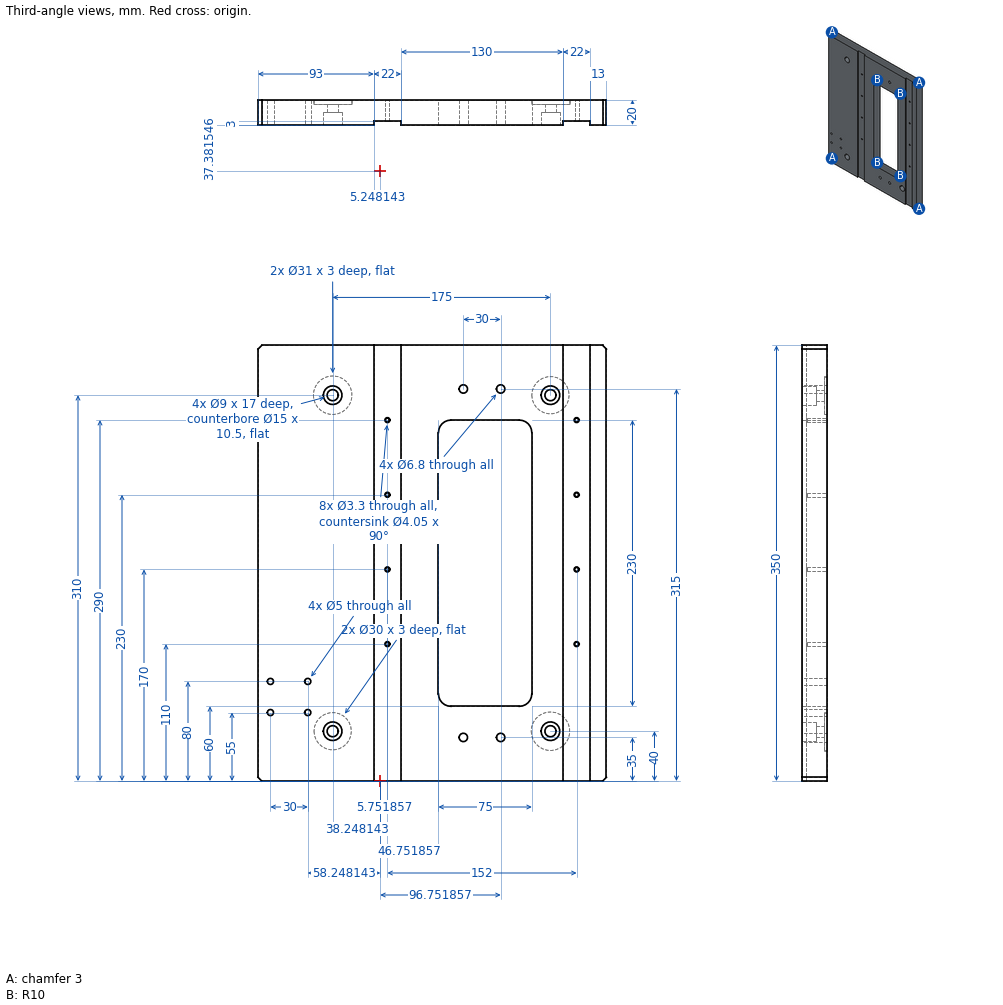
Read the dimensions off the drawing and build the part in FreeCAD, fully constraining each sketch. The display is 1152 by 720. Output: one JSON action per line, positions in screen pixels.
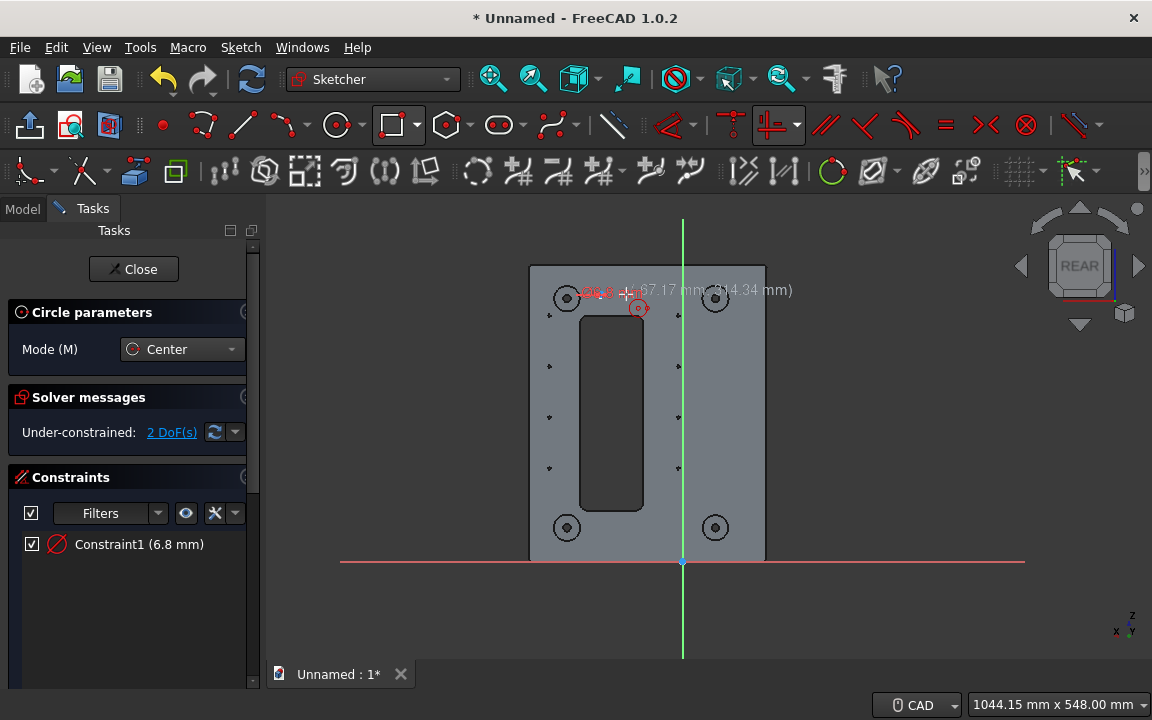
{"action": "left_click", "coordinate": [626, 294]}
{"action": "mouse_move", "coordinate": [628, 292]}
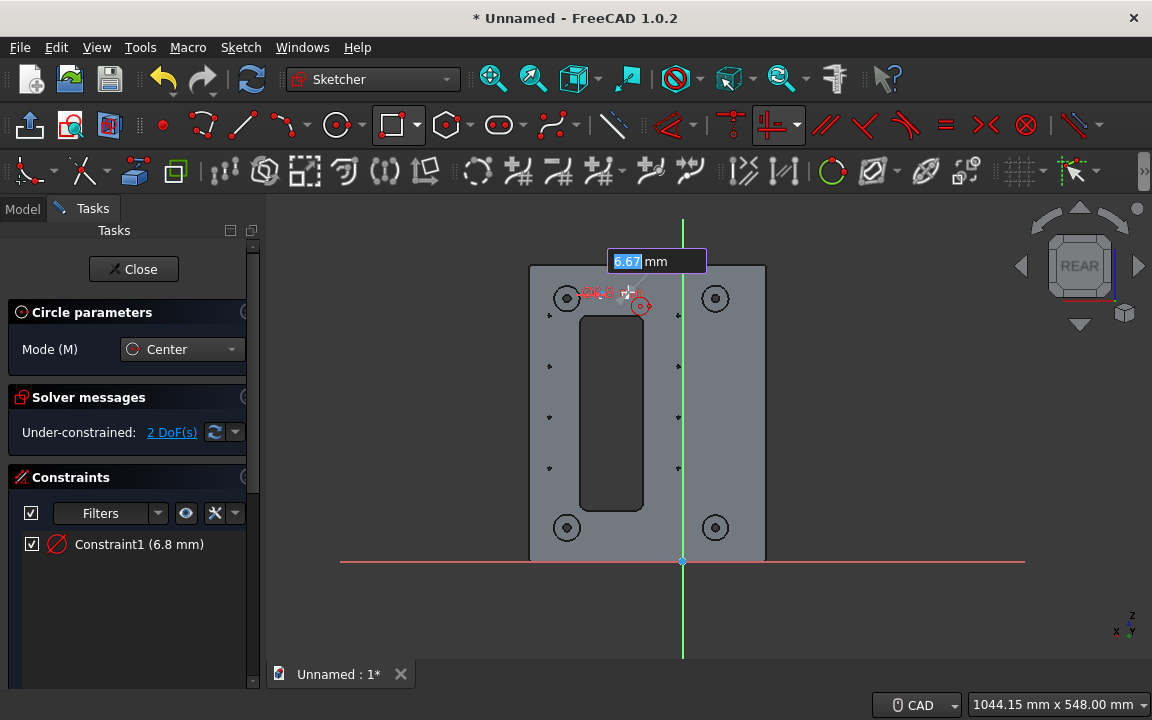
{"action": "type", "text": "6.8"}
{"action": "key", "text": "Return"}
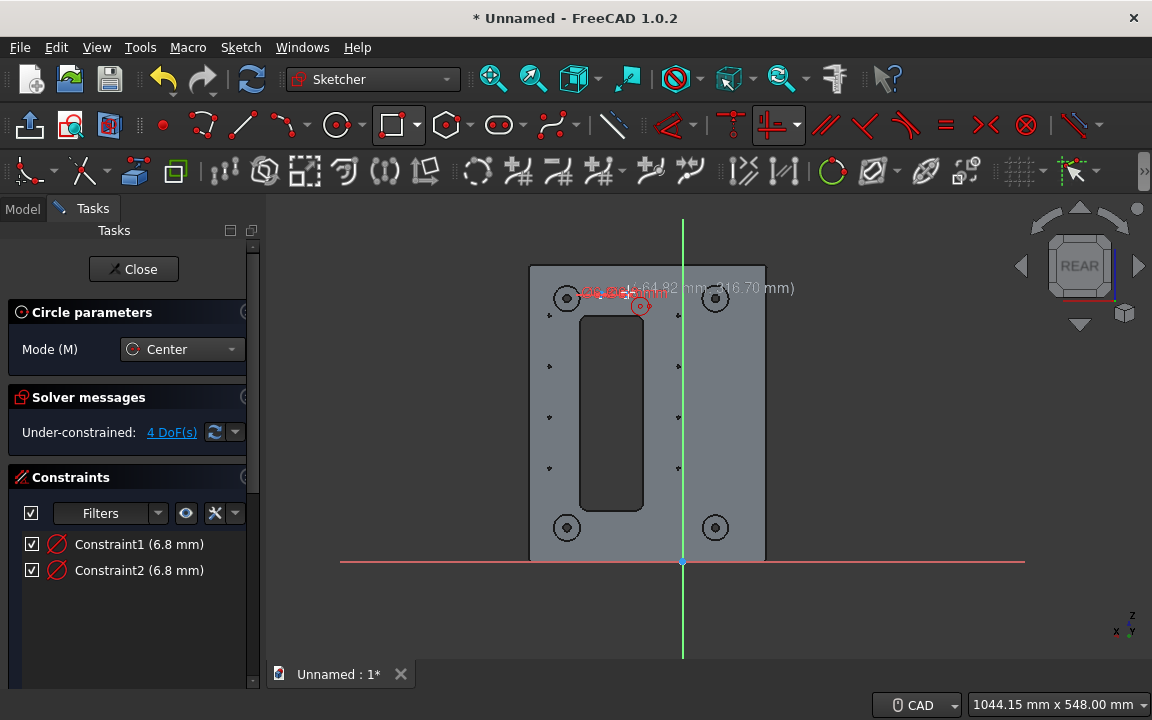
{"action": "scroll", "coordinate": [601, 532], "scroll_direction": "up", "scroll_amount": 11}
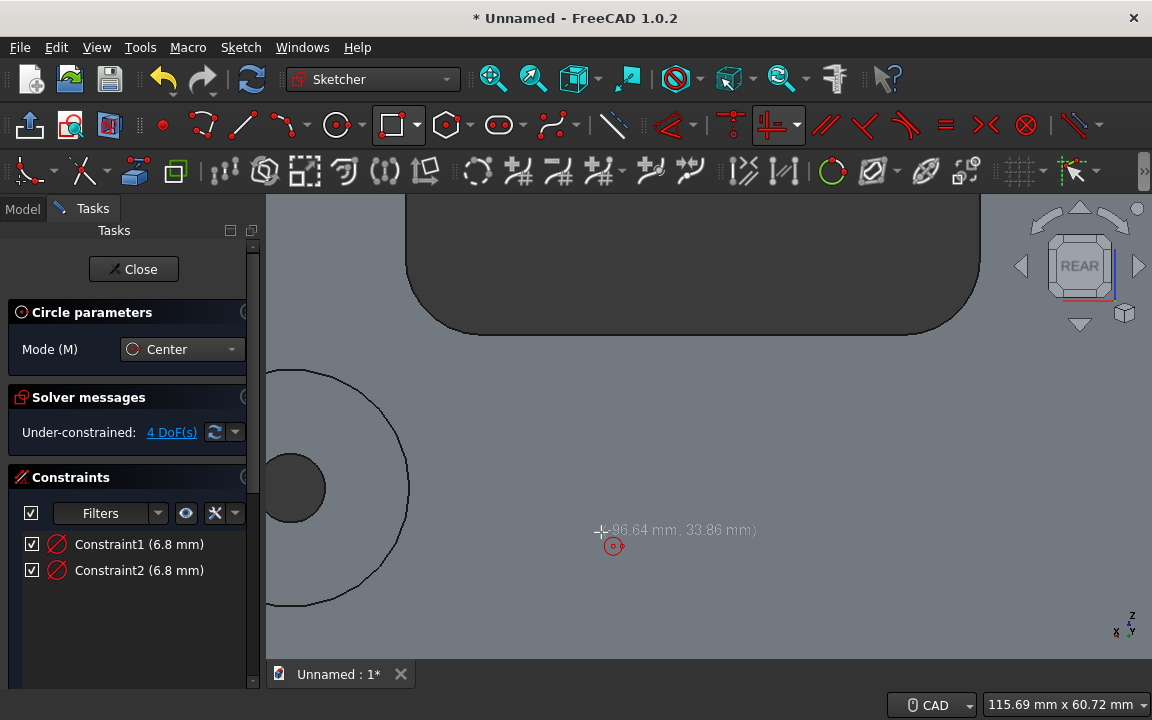
{"action": "scroll", "coordinate": [601, 533], "scroll_direction": "down", "scroll_amount": 11}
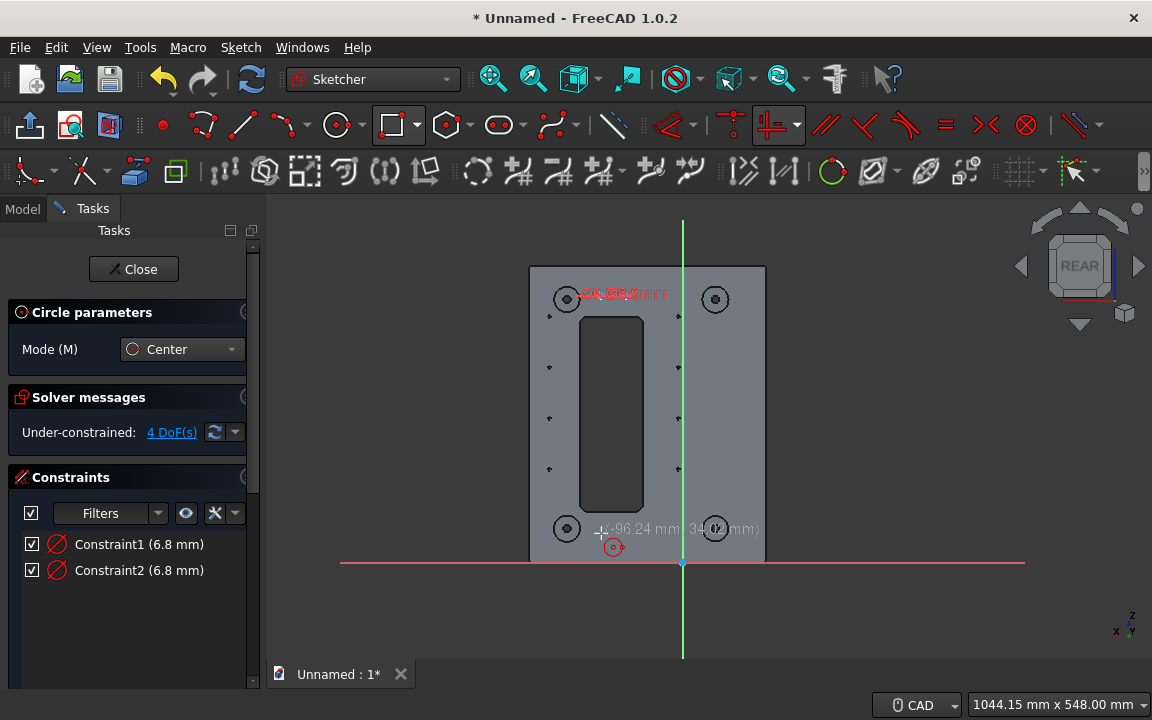
{"action": "left_click", "coordinate": [601, 533]}
{"action": "mouse_move", "coordinate": [603, 531]}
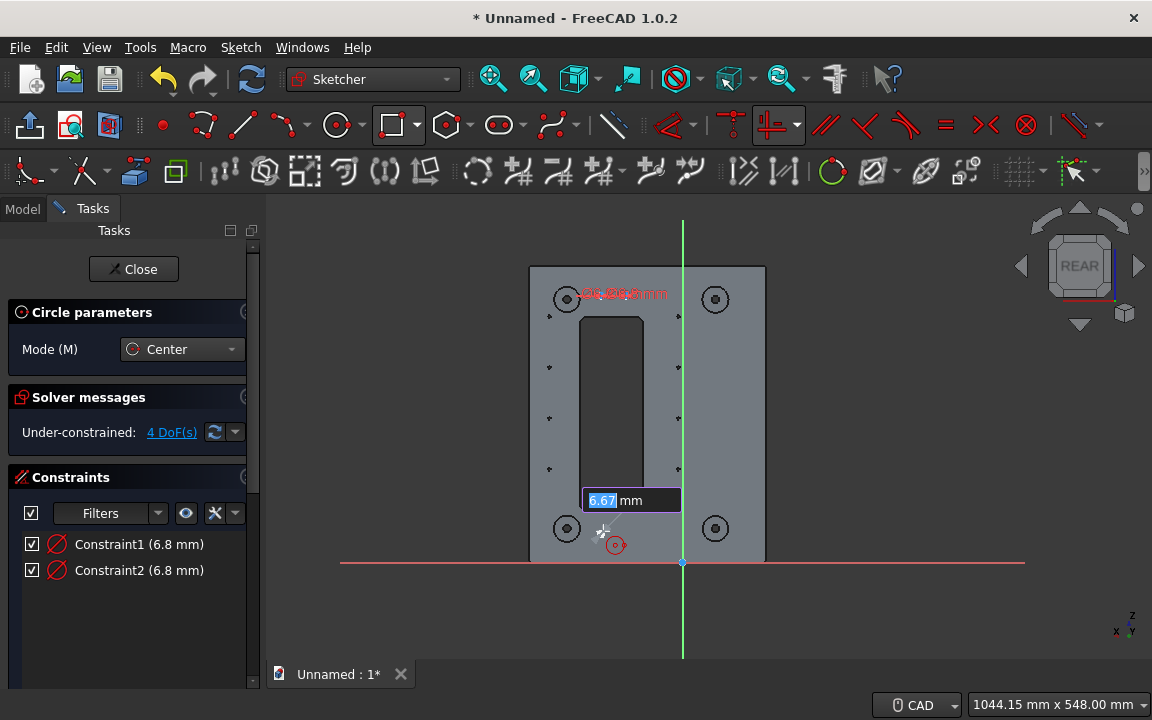
{"action": "type", "text": "6.8"}
{"action": "key", "text": "Return"}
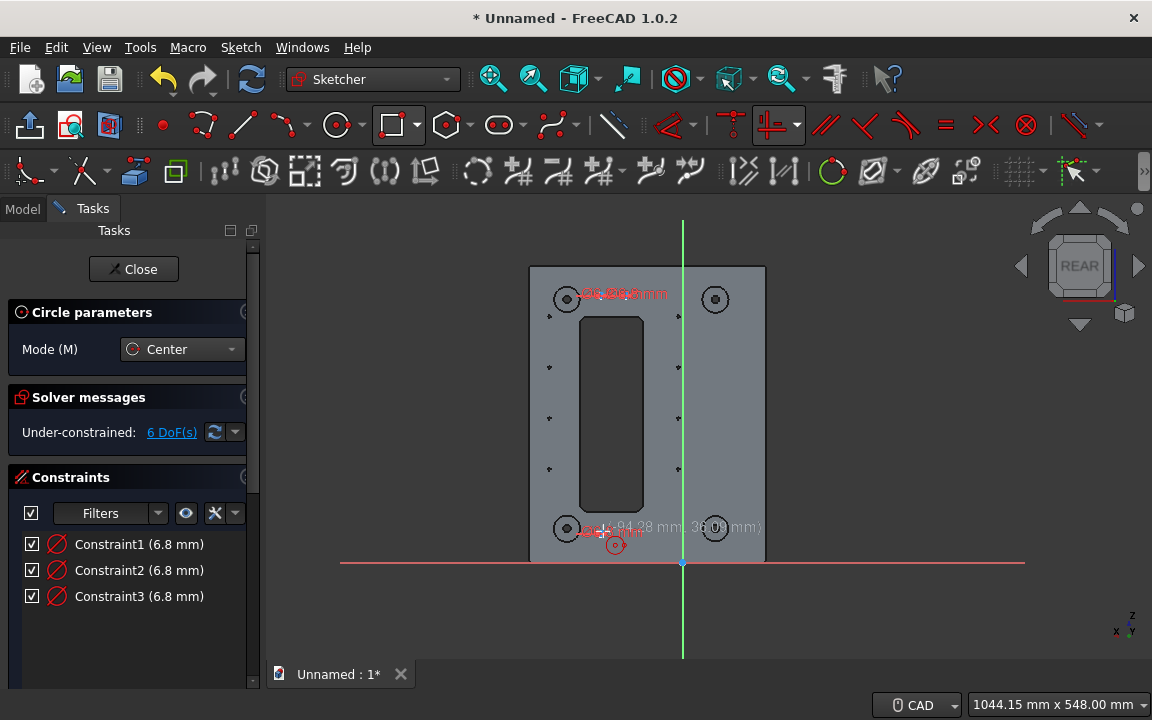
{"action": "scroll", "coordinate": [626, 533], "scroll_direction": "up", "scroll_amount": 11}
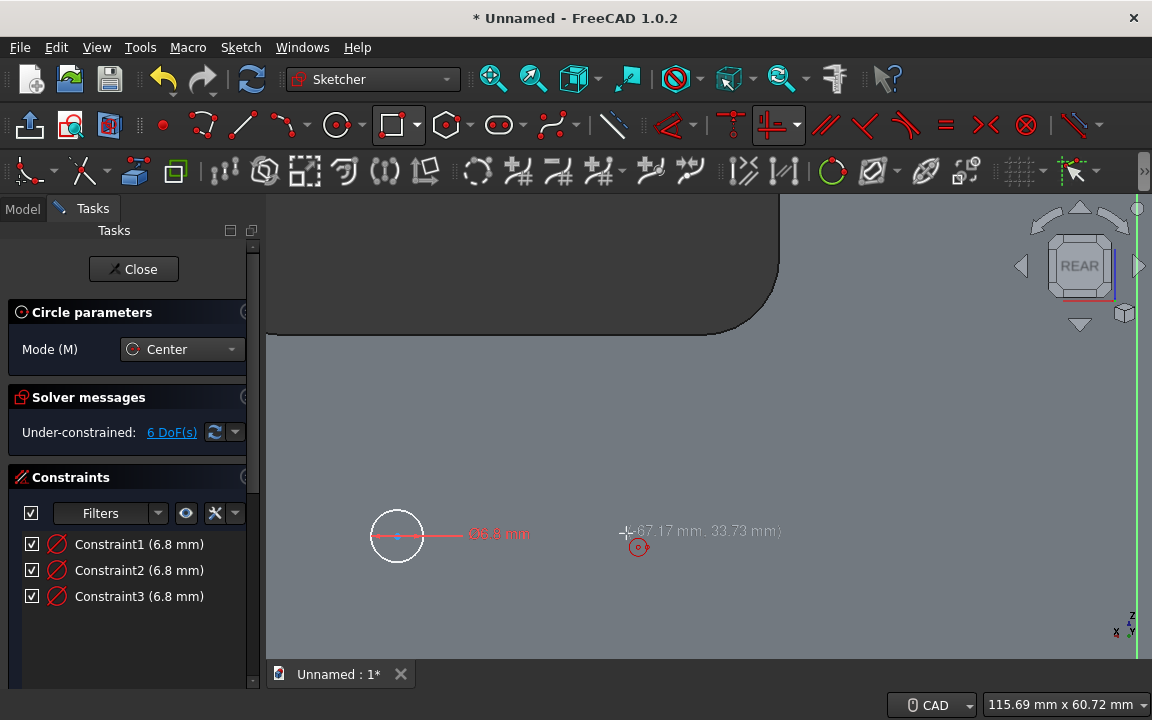
{"action": "scroll", "coordinate": [626, 533], "scroll_direction": "down", "scroll_amount": 11}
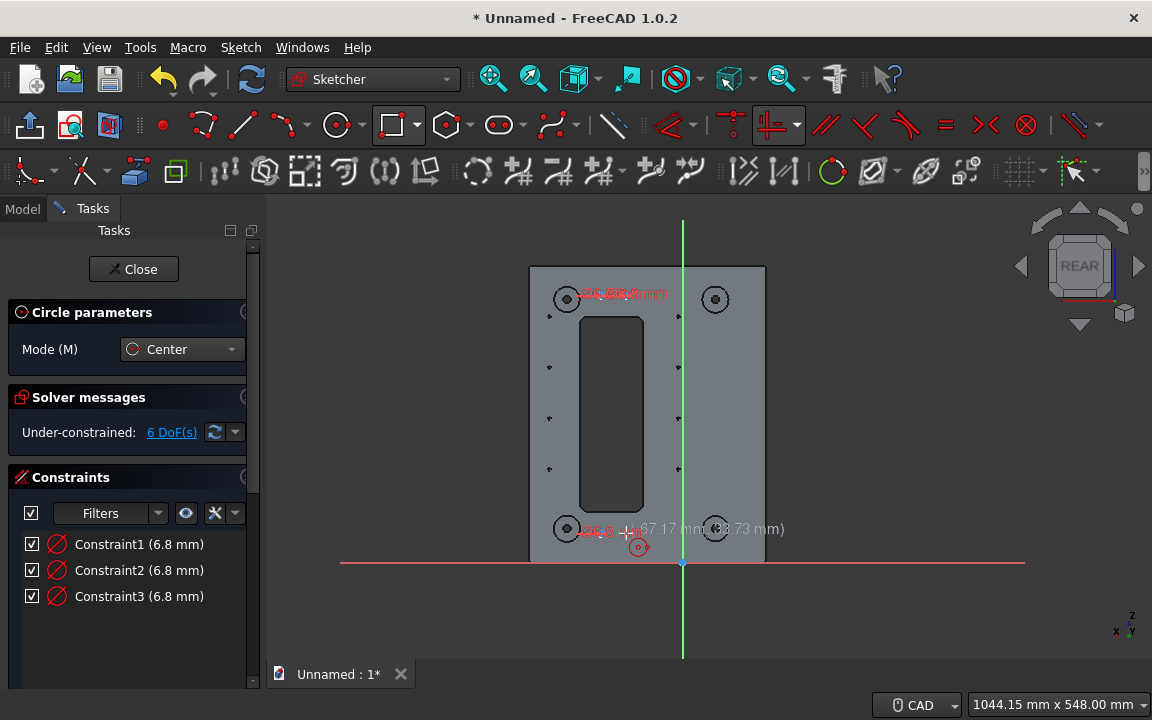
{"action": "left_click", "coordinate": [626, 533]}
{"action": "mouse_move", "coordinate": [628, 531]}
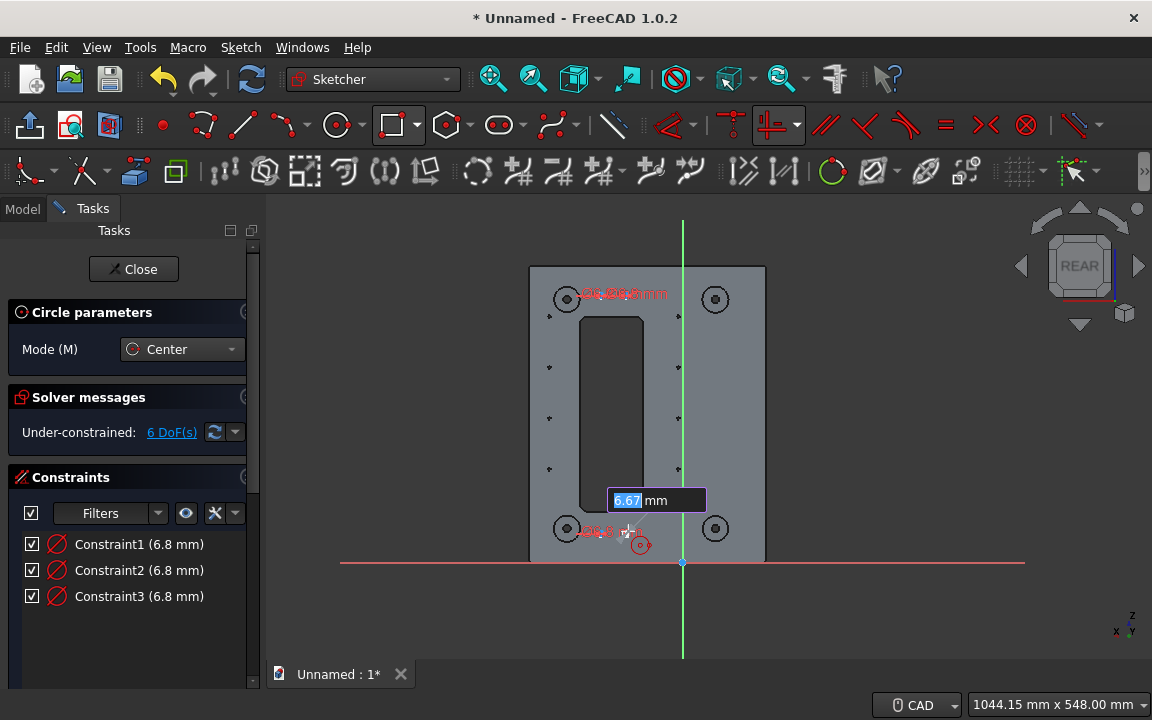
{"action": "type", "text": "6.8"}
{"action": "key", "text": "Return"}
{"action": "key", "text": "Escape"}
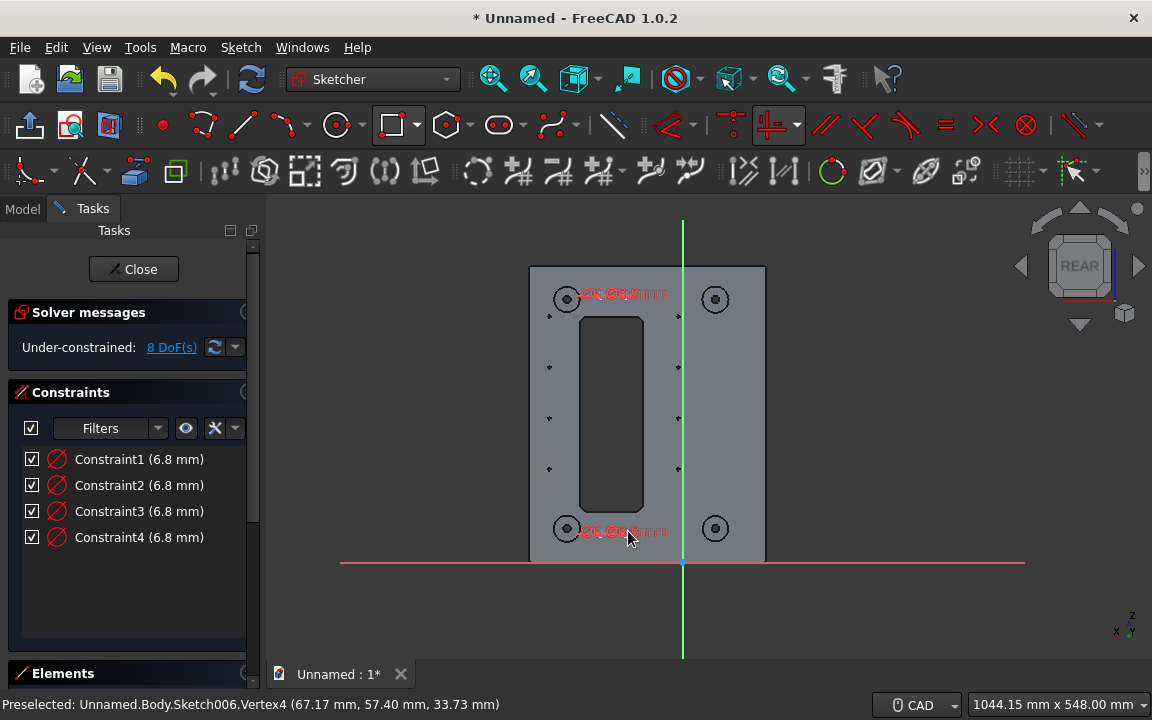
{"action": "left_click", "coordinate": [601, 296]}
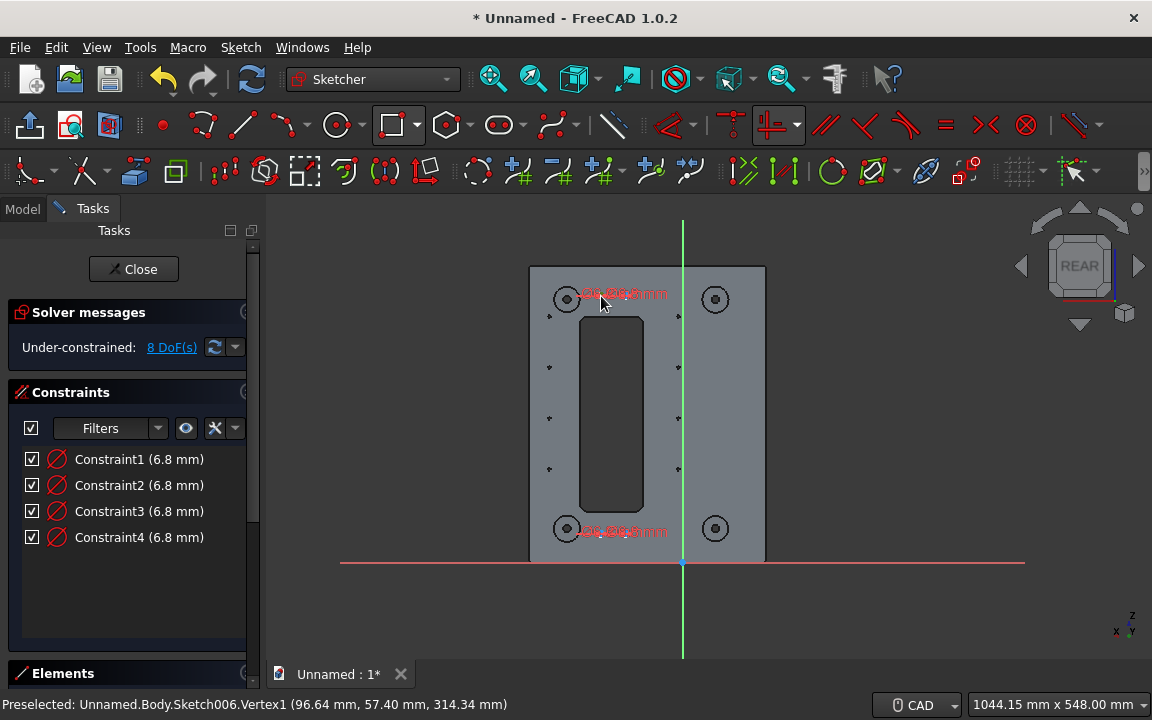
{"action": "left_click", "coordinate": [626, 296]}